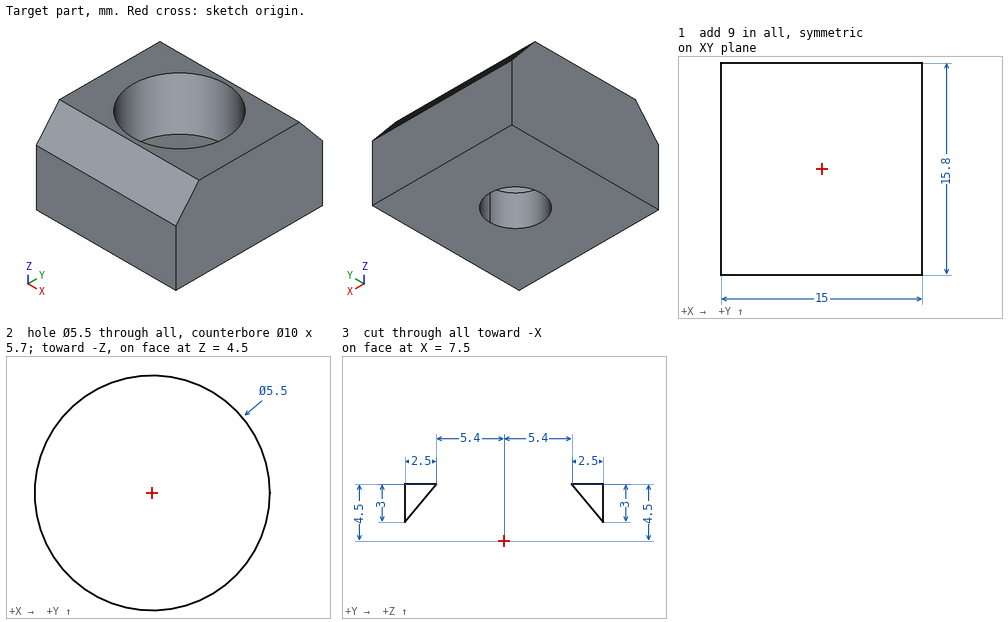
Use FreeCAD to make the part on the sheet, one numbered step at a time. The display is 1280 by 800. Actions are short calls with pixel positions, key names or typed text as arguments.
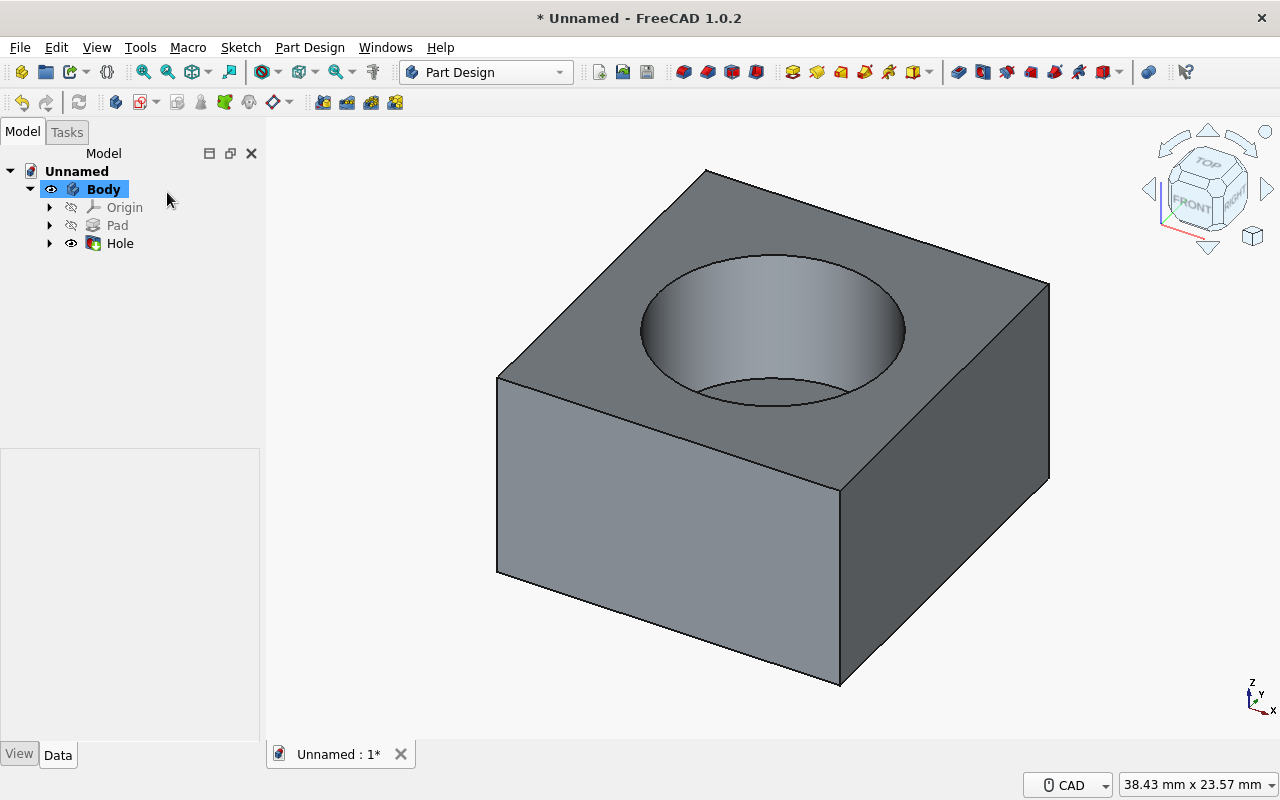
click(974, 454)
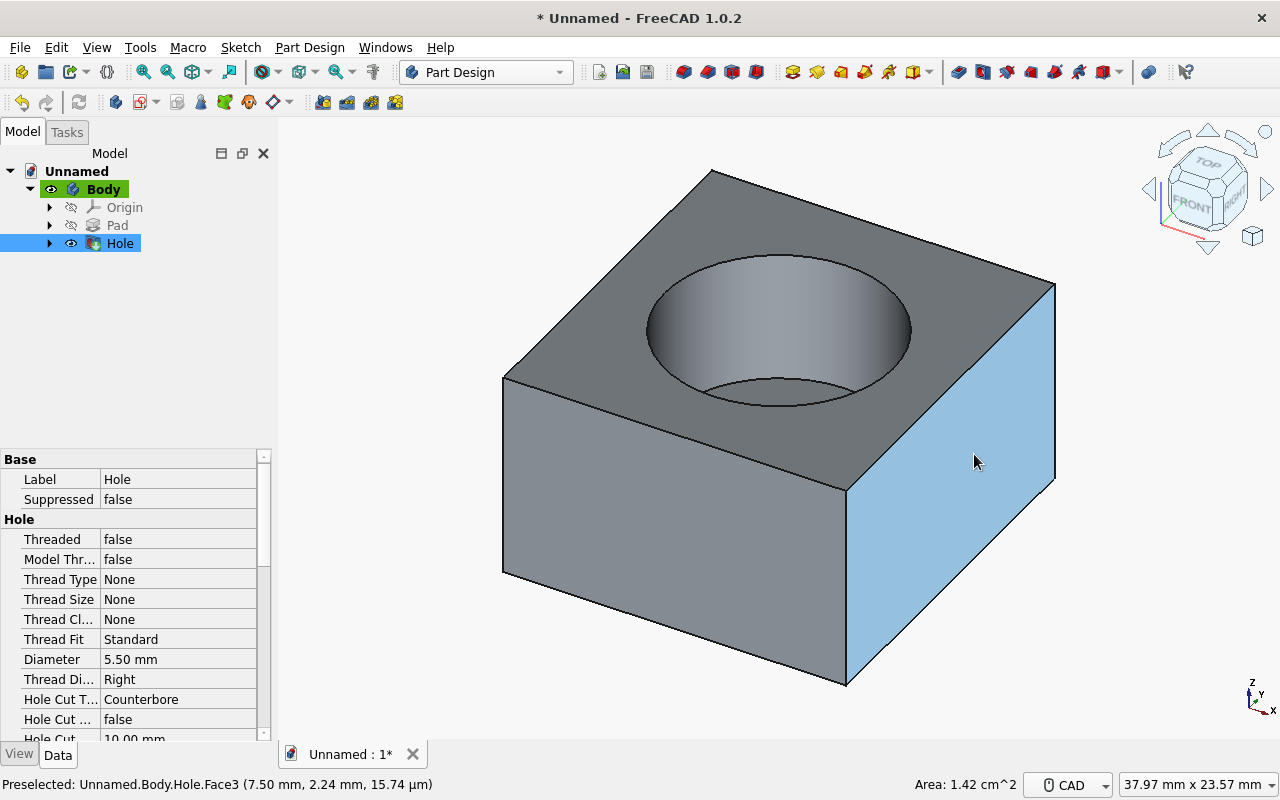
click(140, 102)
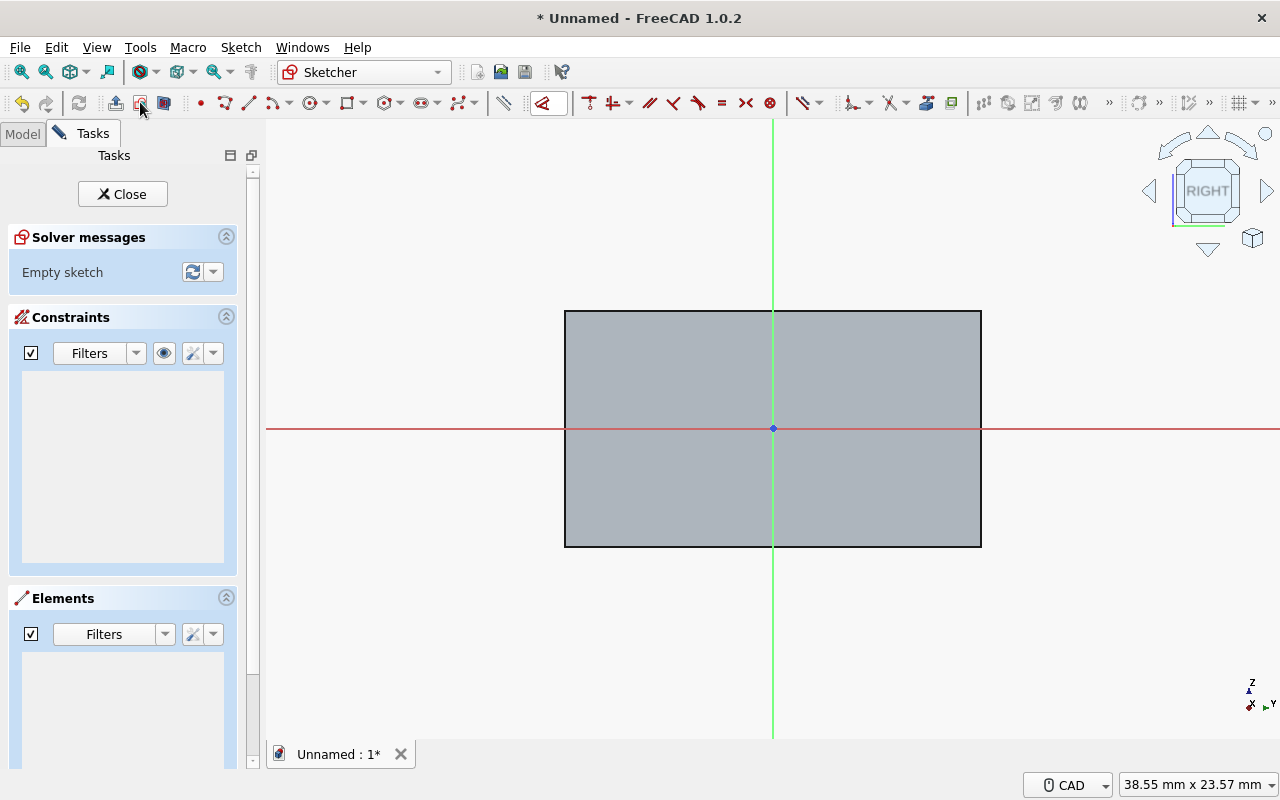
scroll(912, 249, up, 2)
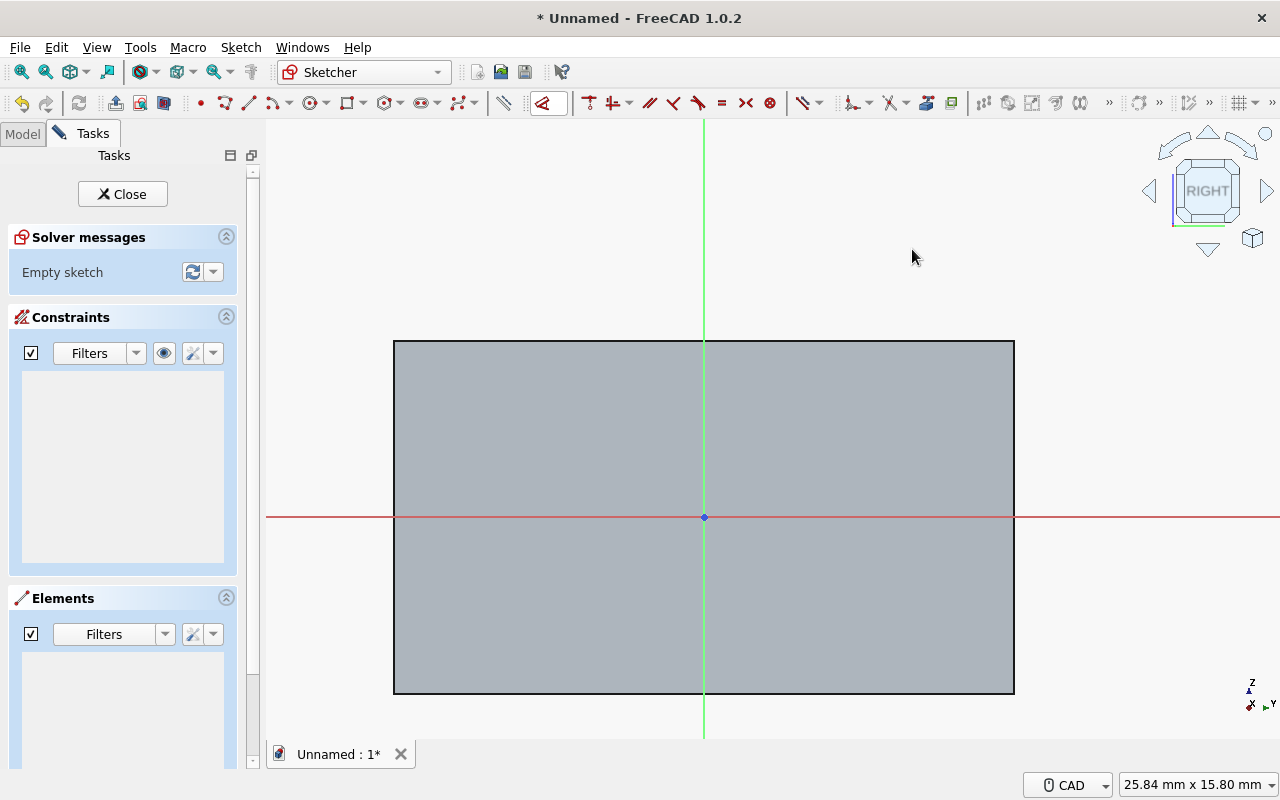
click(226, 104)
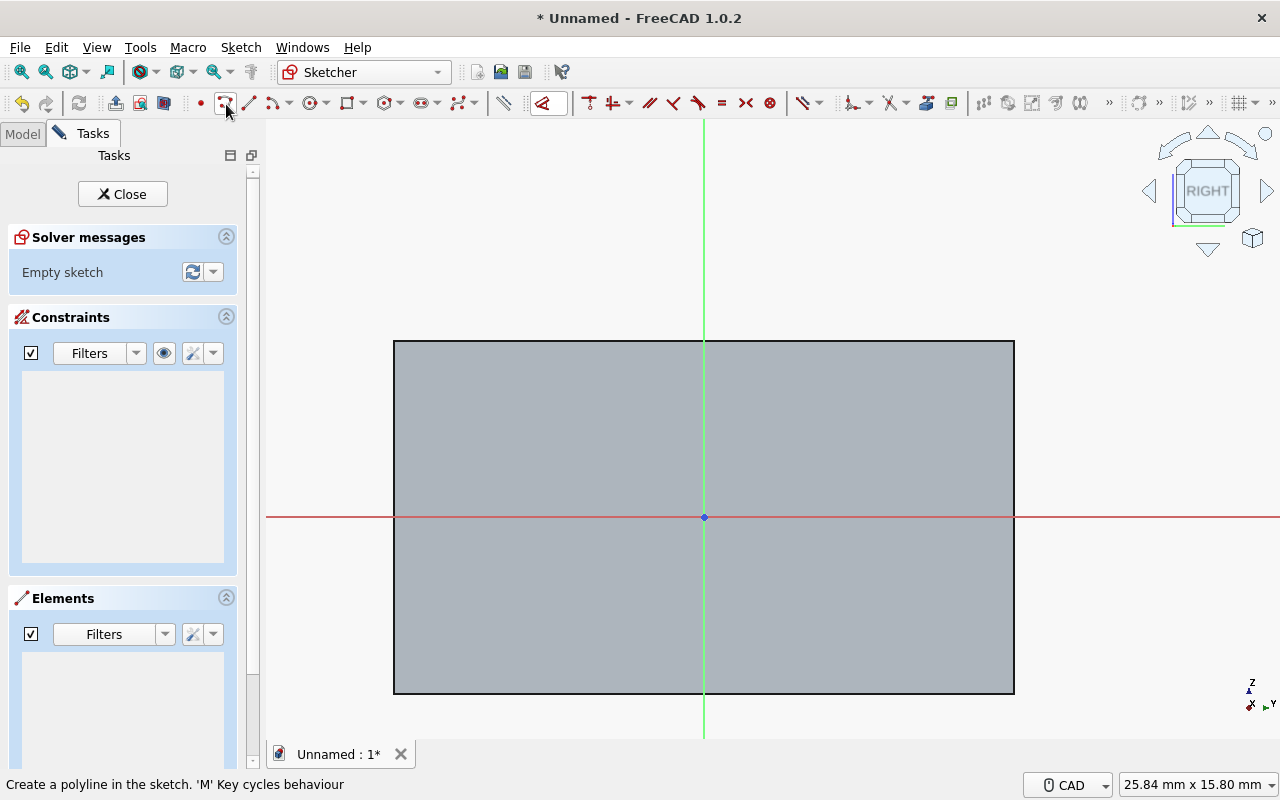
click(492, 341)
click(394, 341)
click(394, 459)
click(492, 342)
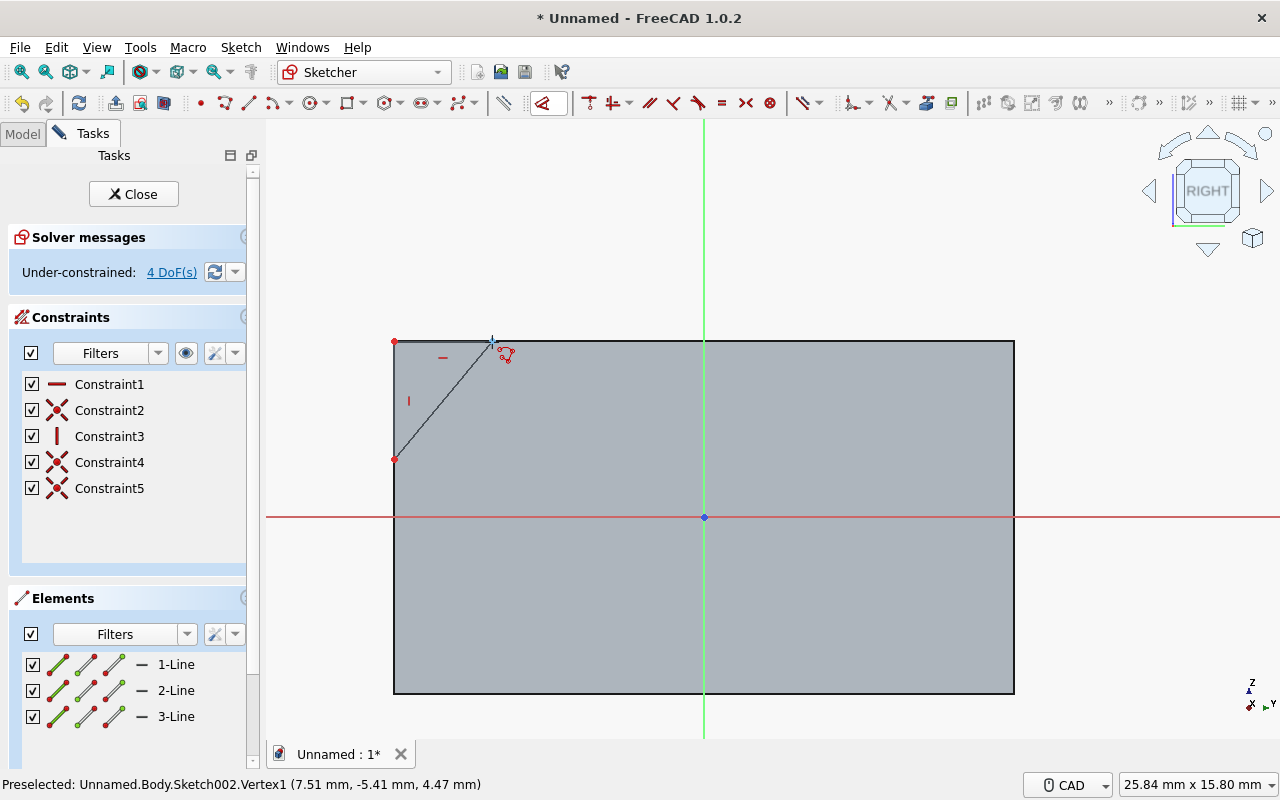
click(916, 341)
click(1014, 459)
click(1014, 341)
click(916, 342)
key(Escape)
key(Escape)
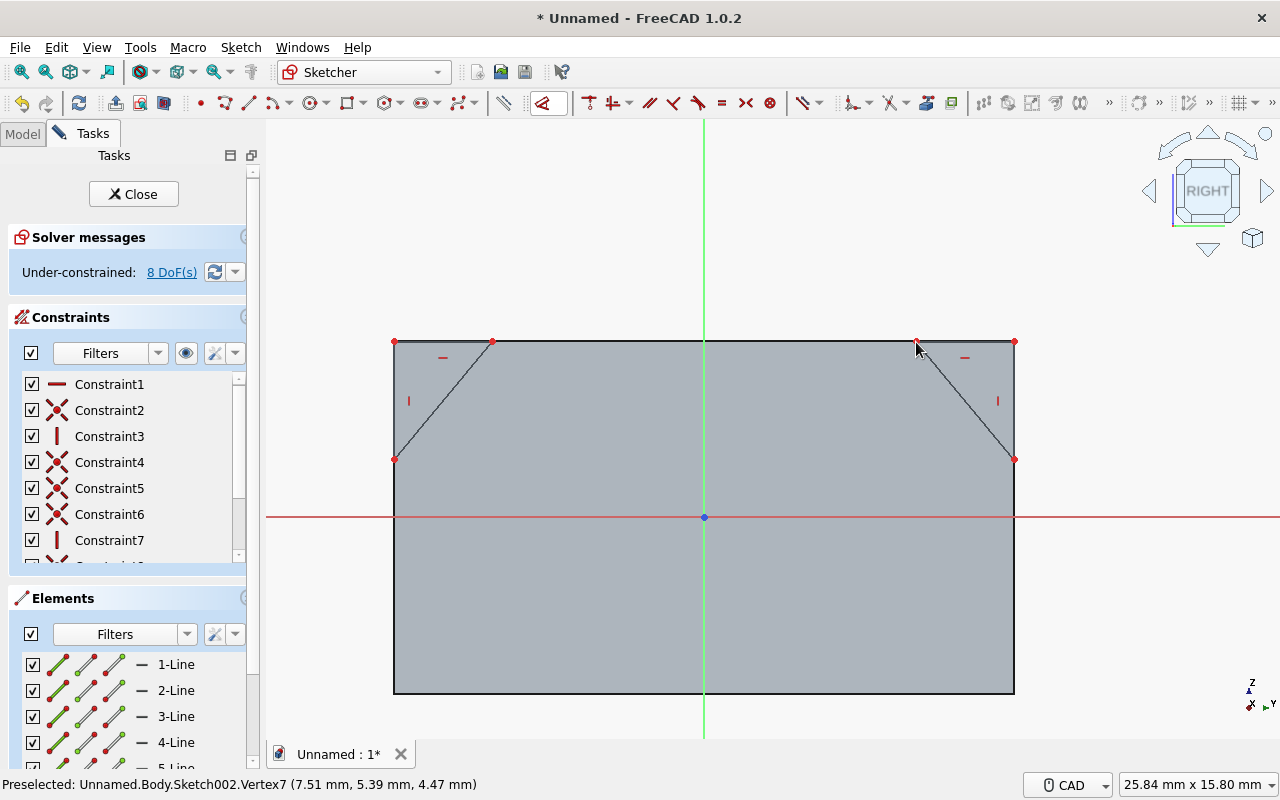
click(394, 377)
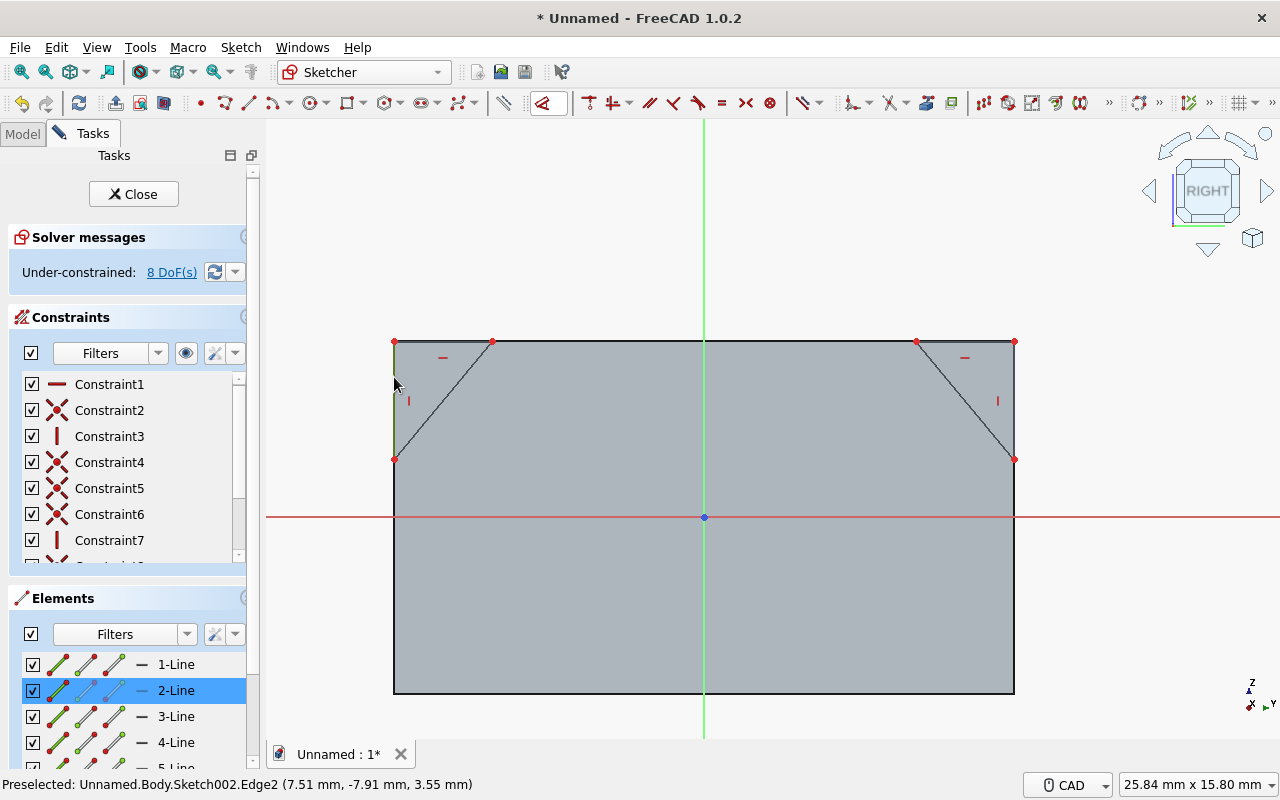
key(i)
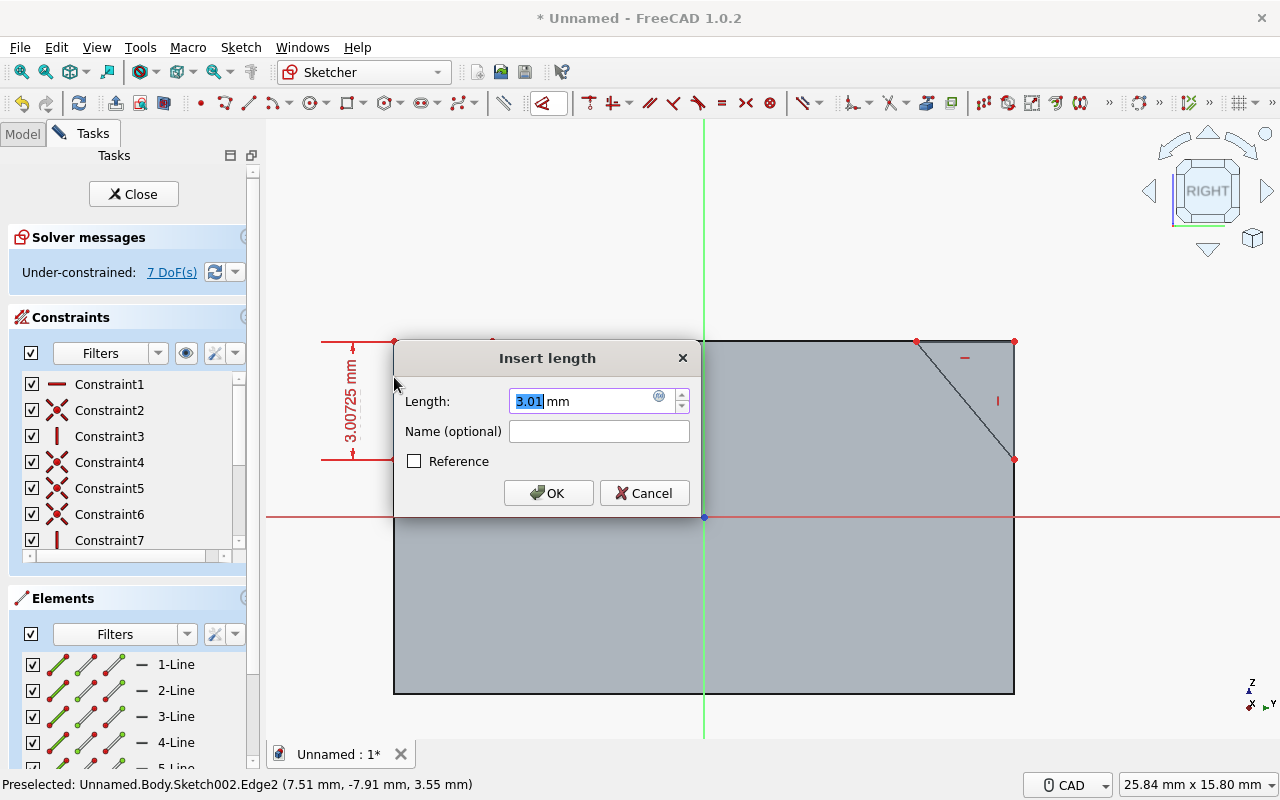
text(3)
key(Return)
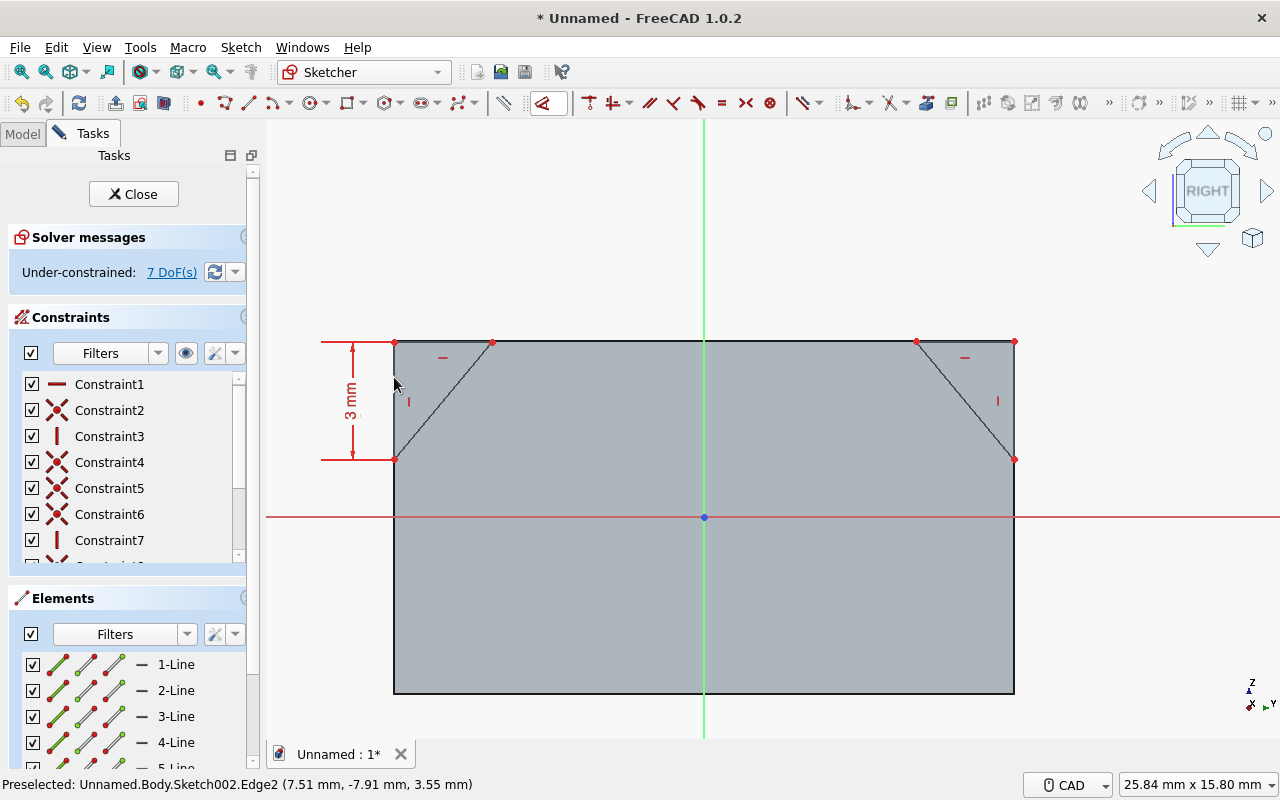
click(1014, 425)